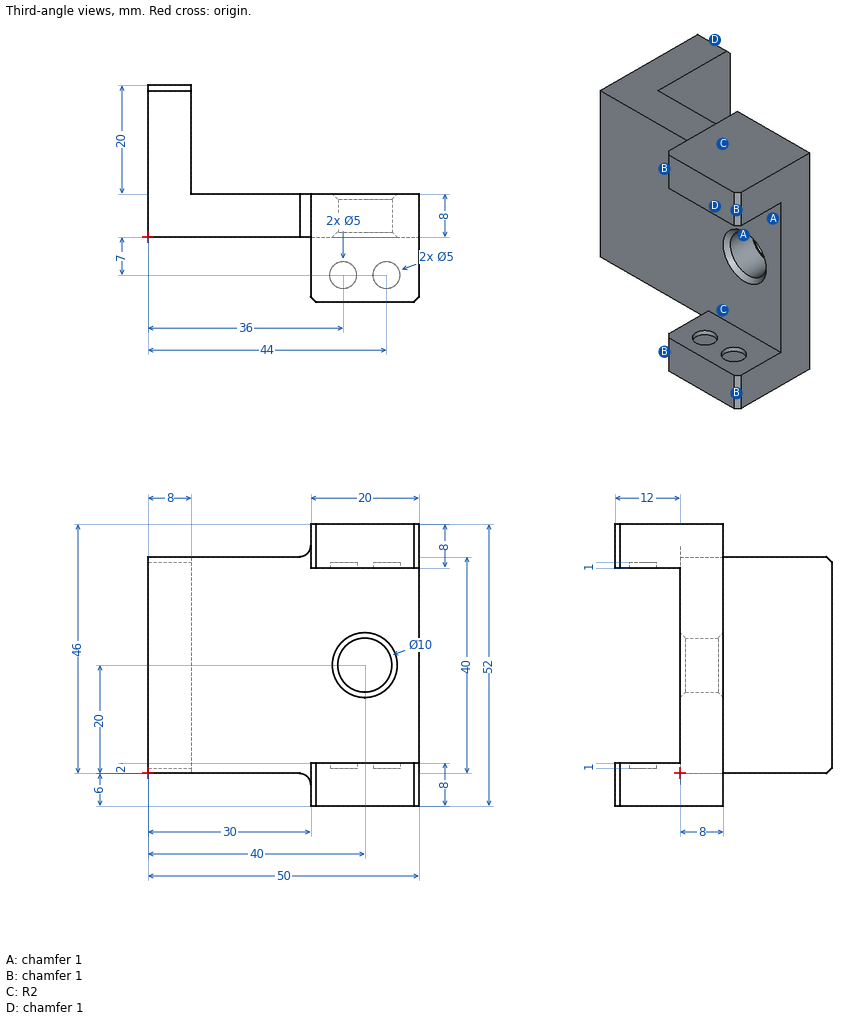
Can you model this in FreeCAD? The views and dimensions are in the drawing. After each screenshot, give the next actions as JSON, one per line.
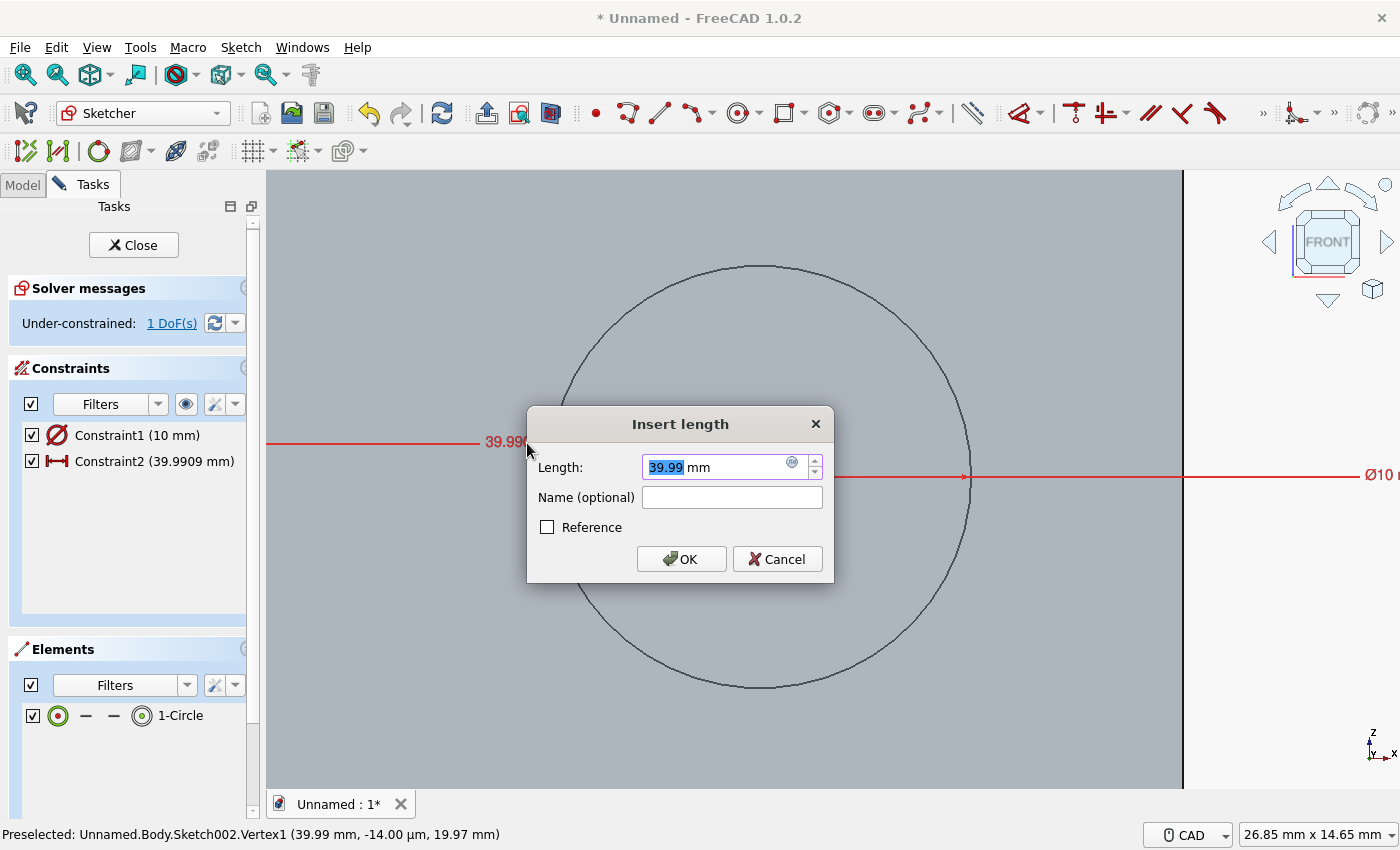
{"action": "type", "text": "40"}
{"action": "key", "text": "Return"}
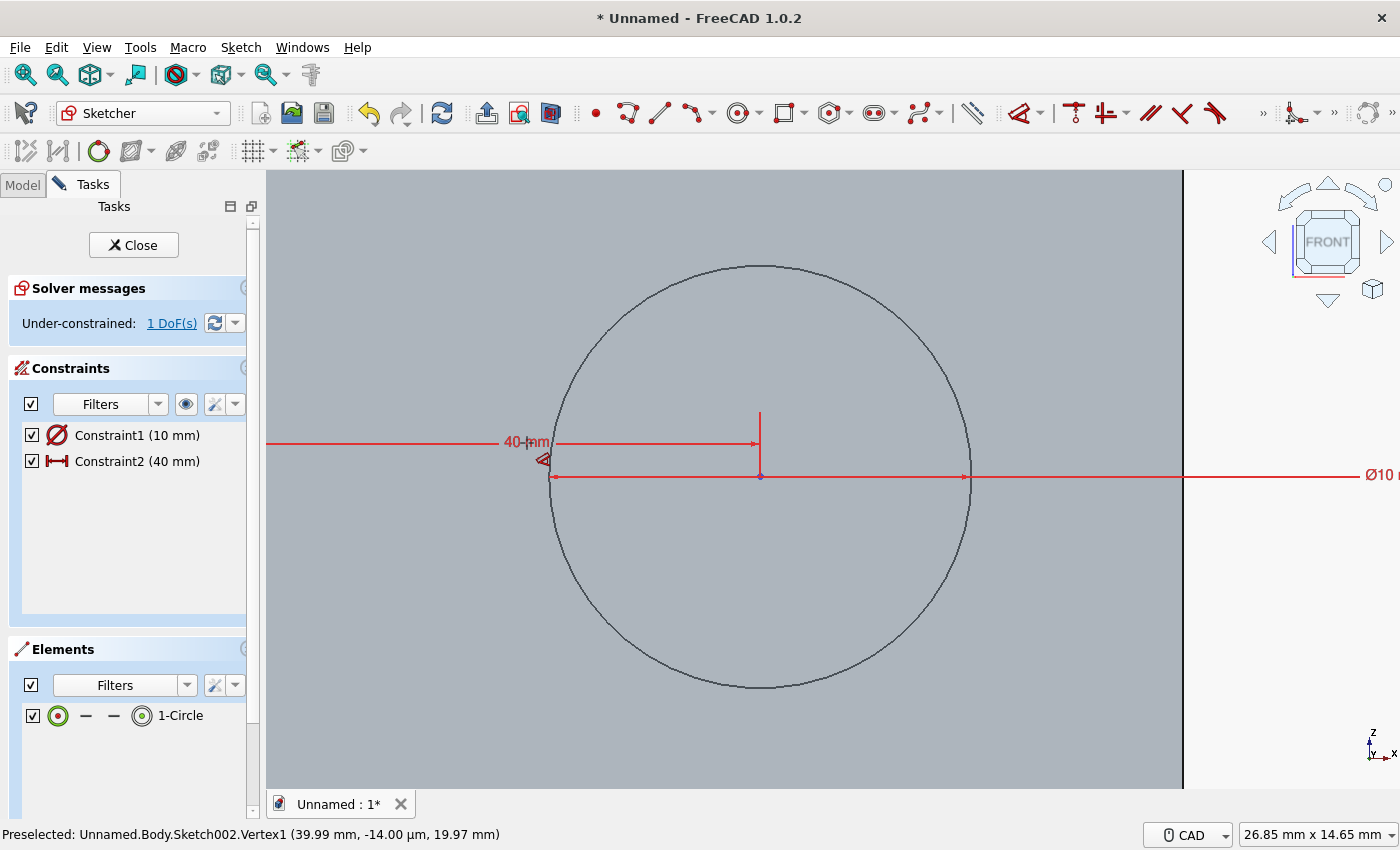
{"action": "left_click", "coordinate": [760, 477]}
{"action": "left_click", "coordinate": [794, 619]}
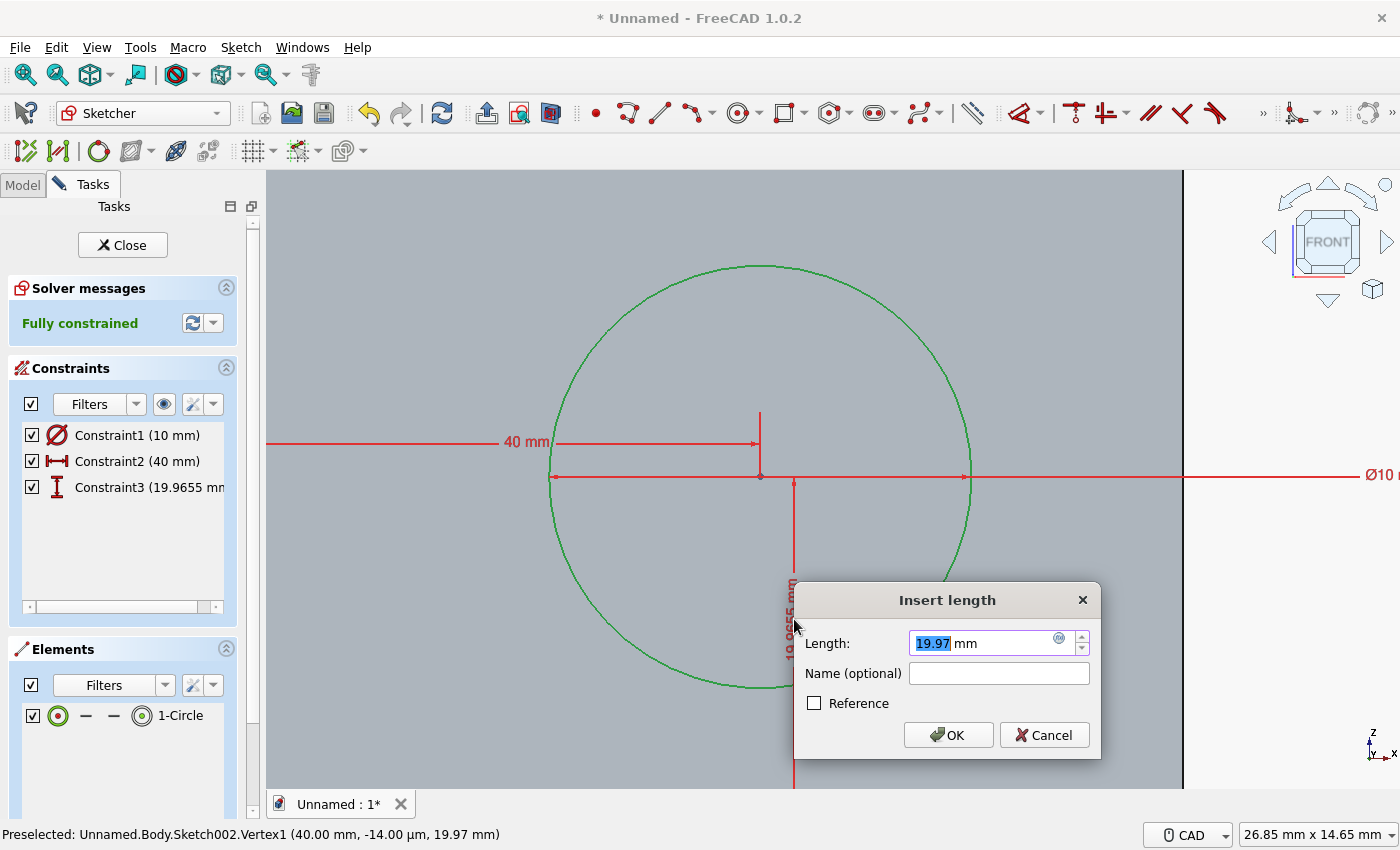
{"action": "type", "text": "20"}
{"action": "key", "text": "Return"}
{"action": "key", "text": "Escape"}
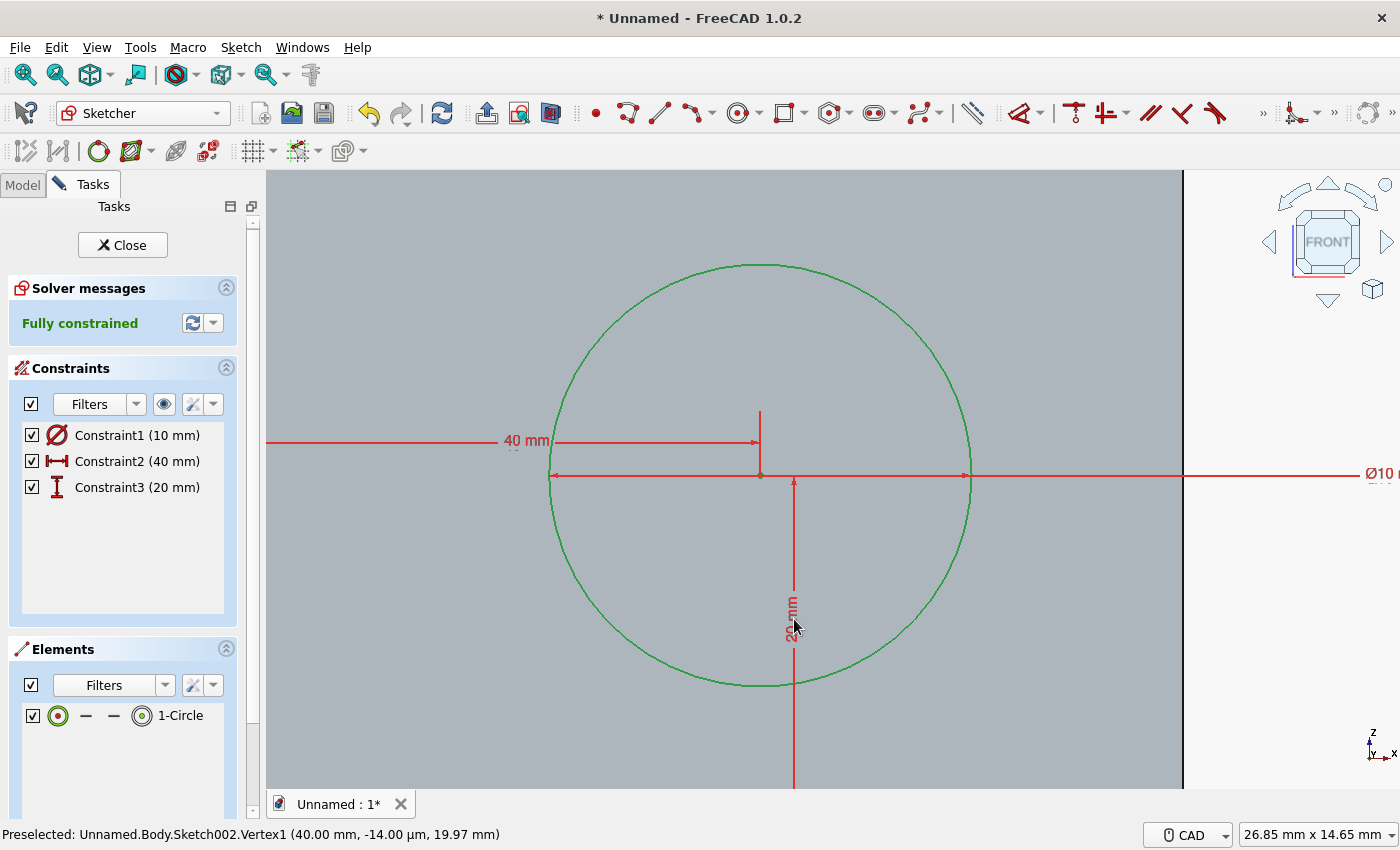
{"action": "left_click", "coordinate": [123, 245]}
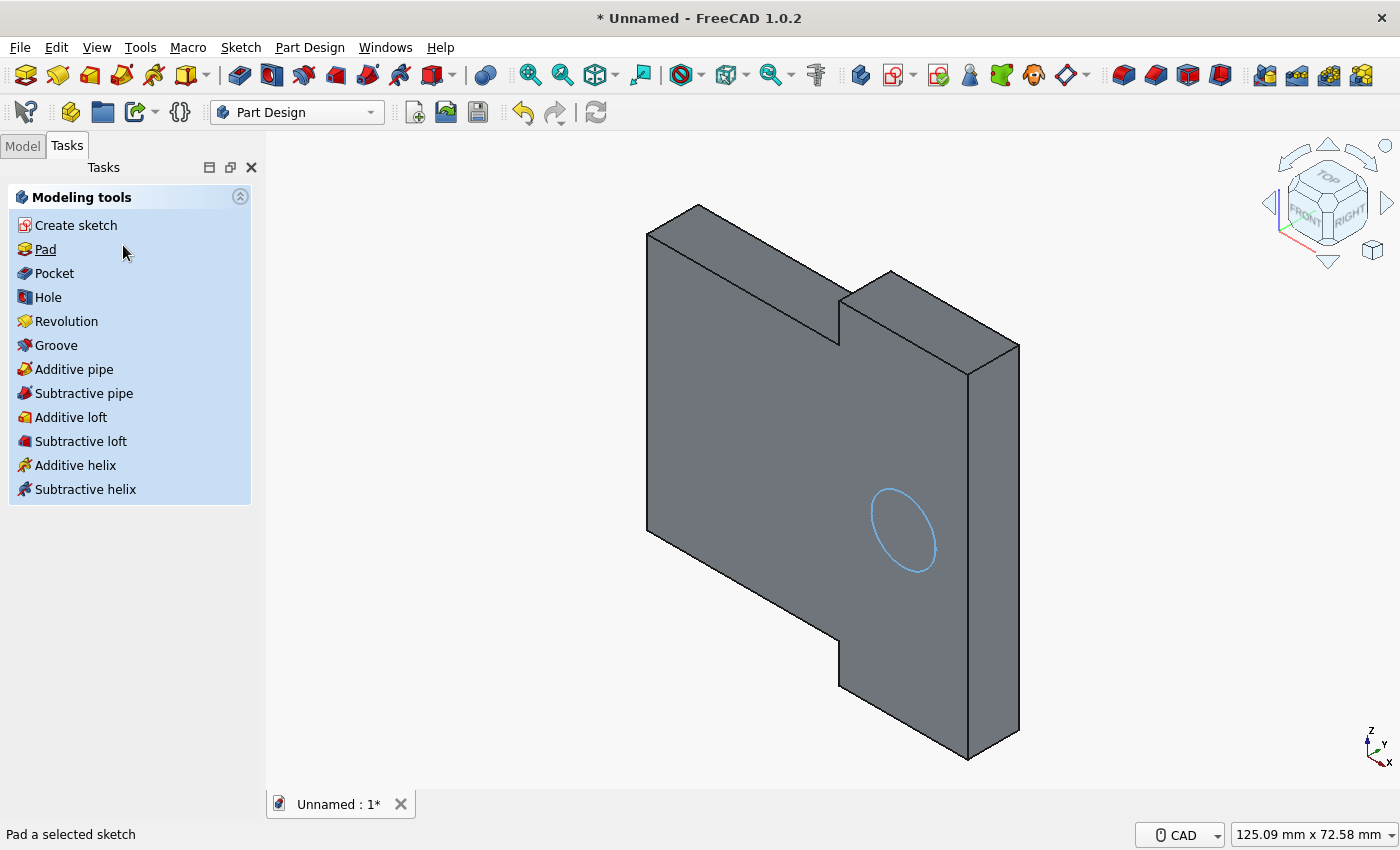
{"action": "left_click", "coordinate": [240, 76]}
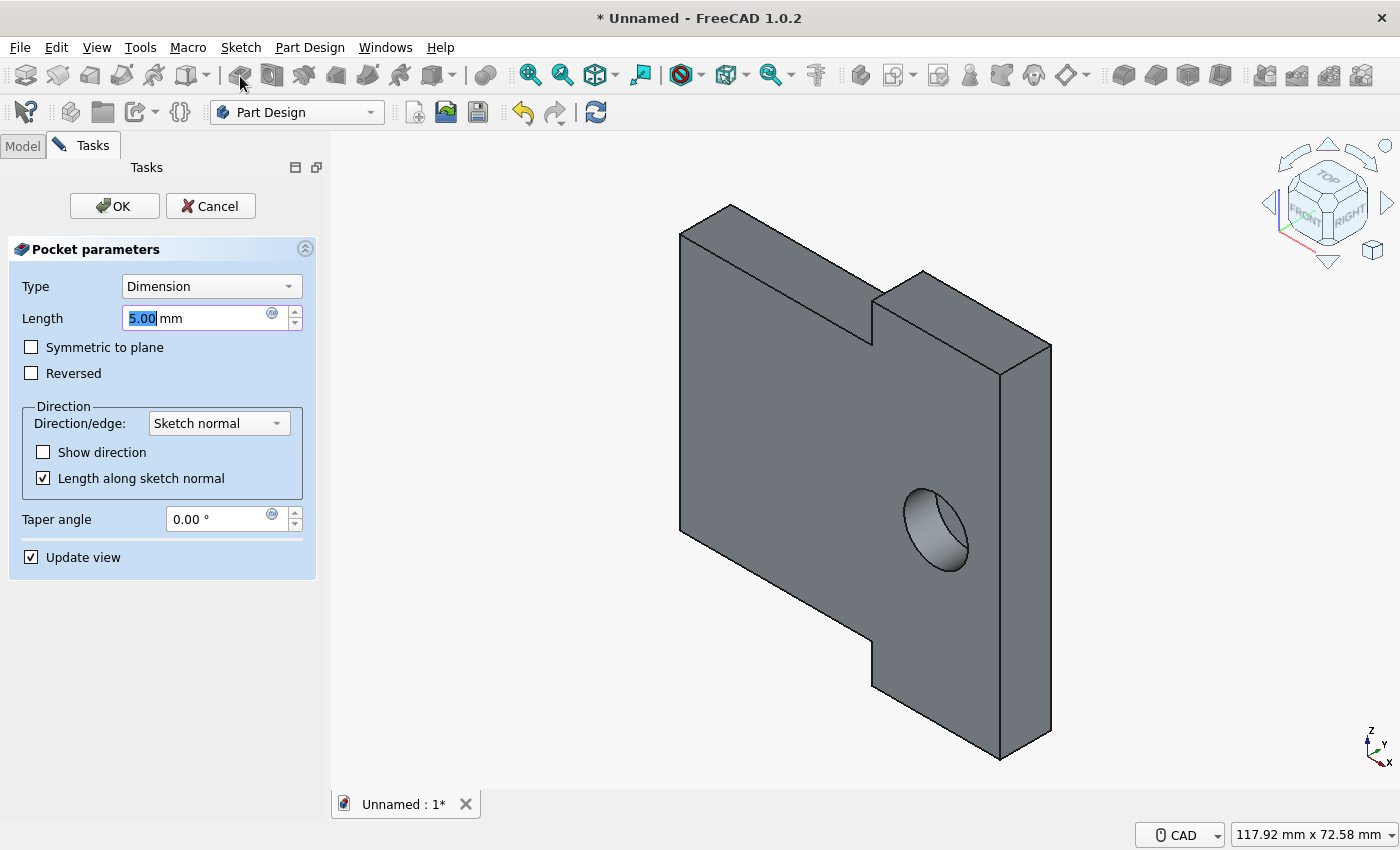
{"action": "left_click", "coordinate": [212, 286]}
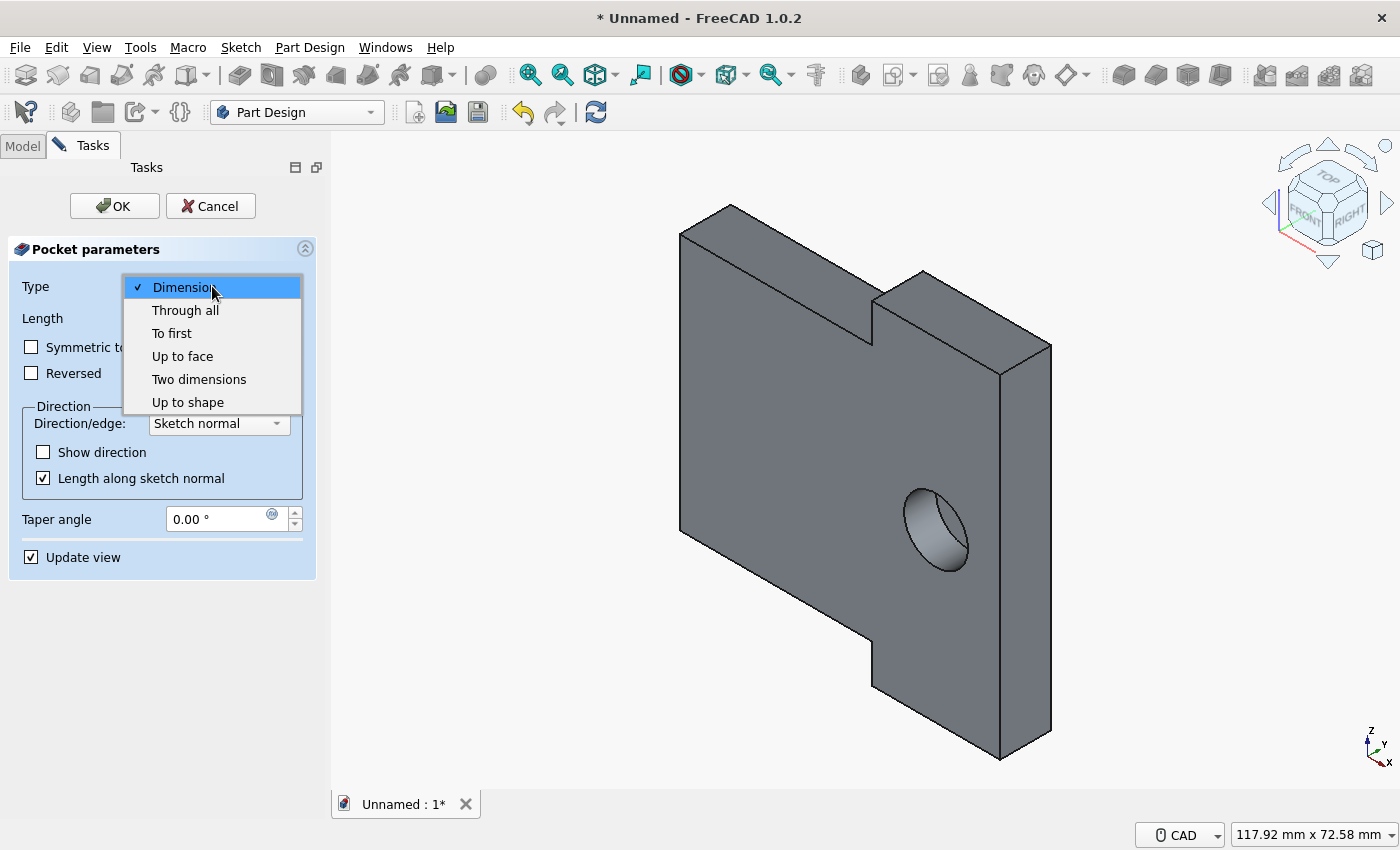
{"action": "left_click", "coordinate": [212, 310]}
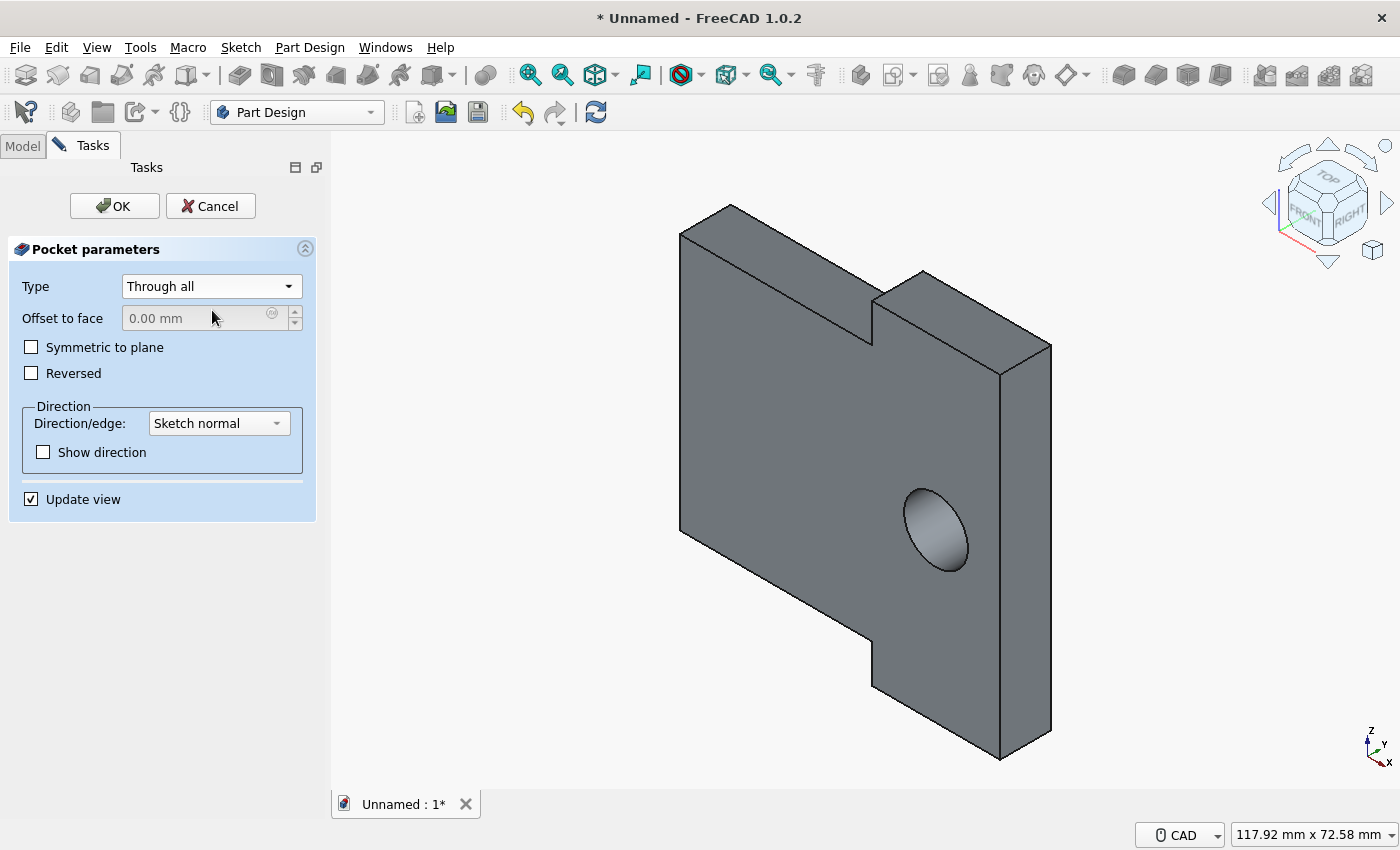
{"action": "left_click", "coordinate": [115, 206]}